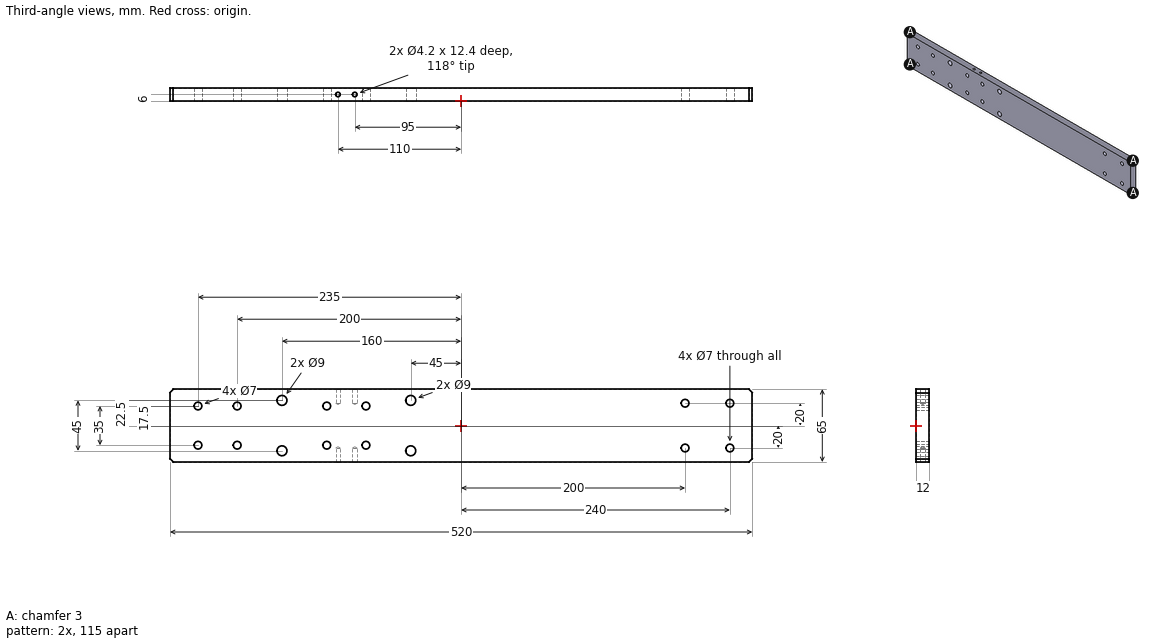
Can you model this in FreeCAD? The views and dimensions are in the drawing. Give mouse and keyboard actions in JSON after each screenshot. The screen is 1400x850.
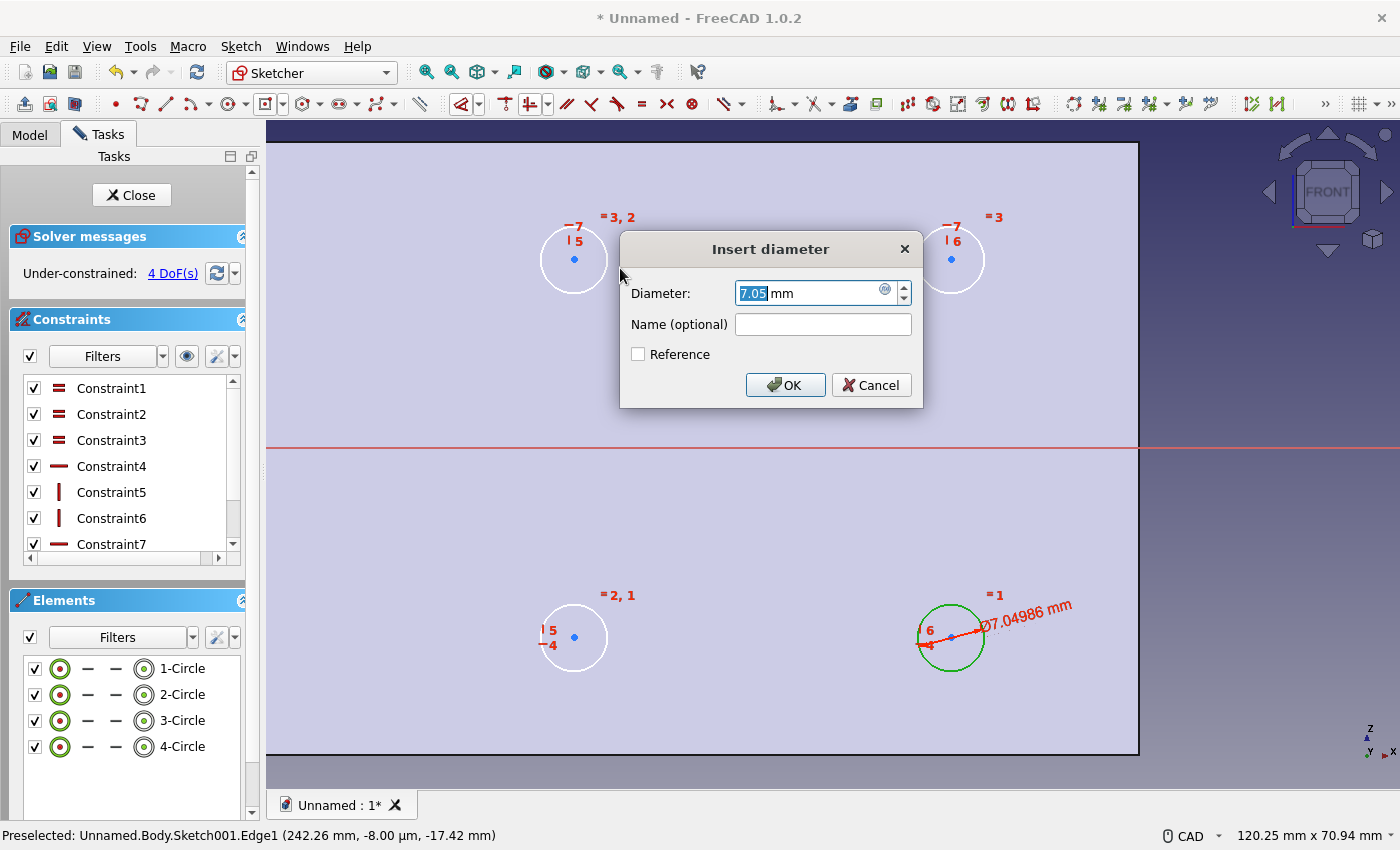
{"action": "type", "text": "7"}
{"action": "key", "text": "Return"}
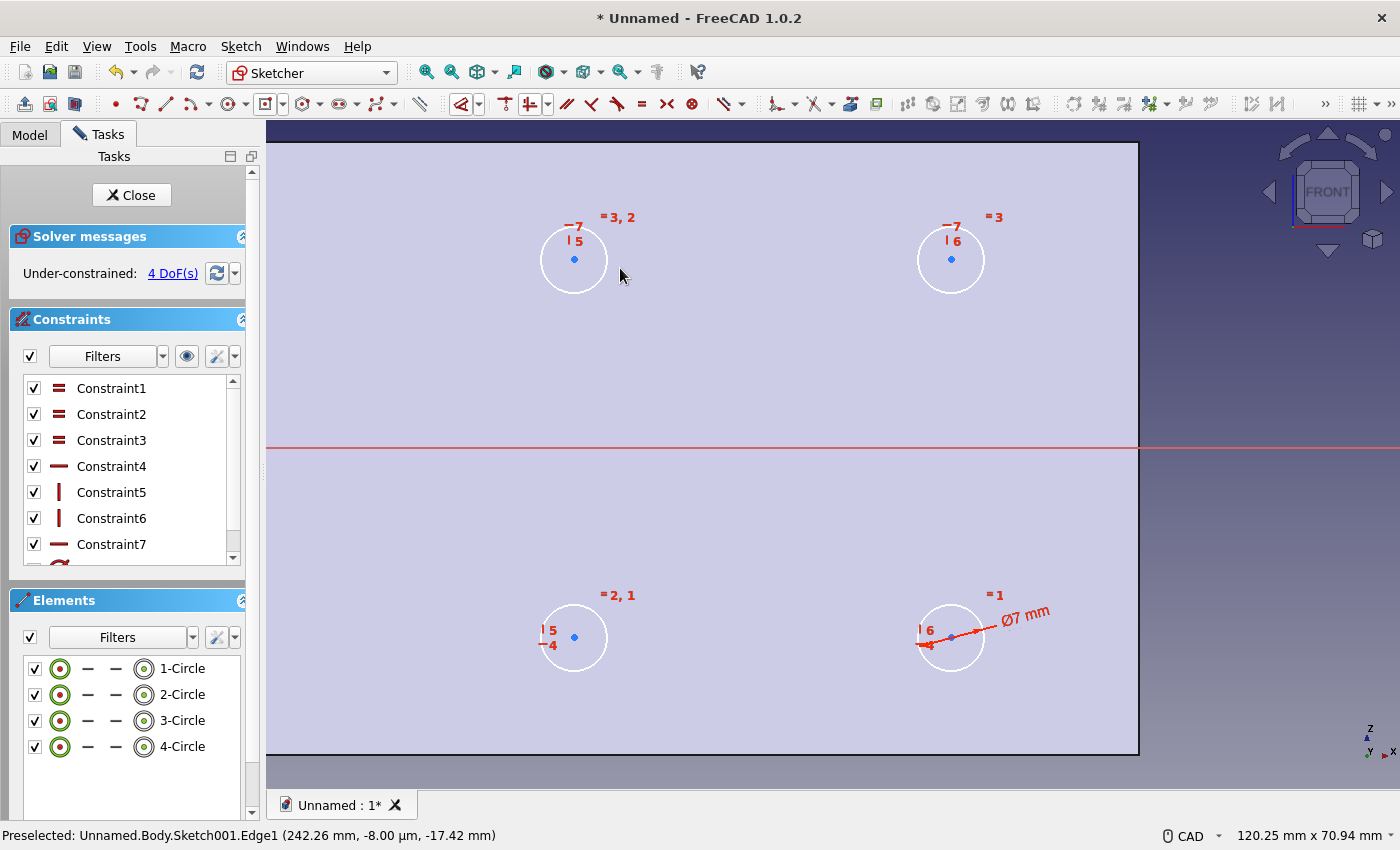
{"action": "left_click", "coordinate": [951, 638]}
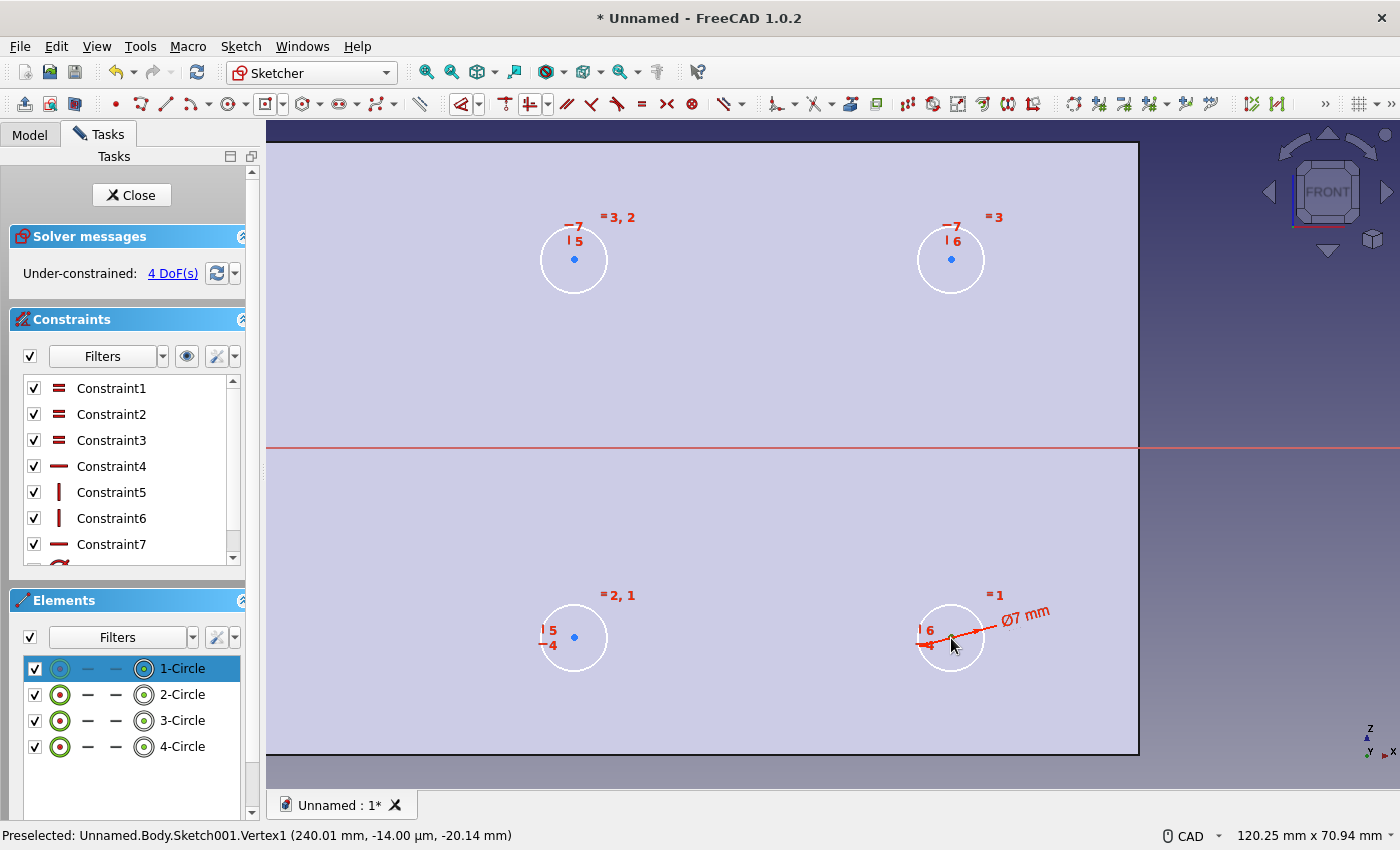
{"action": "key", "text": "i"}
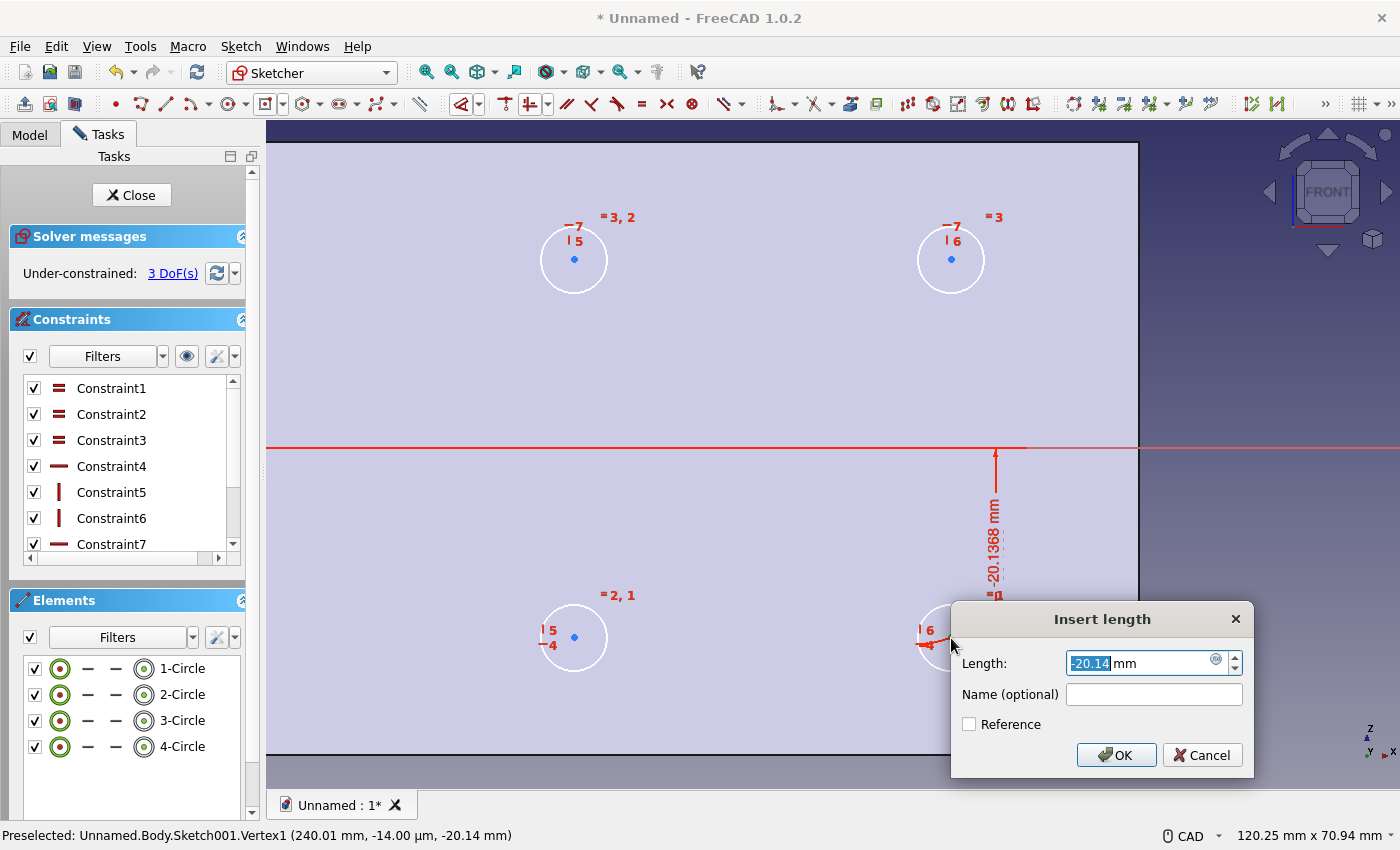
{"action": "type", "text": "-20"}
{"action": "key", "text": "Return"}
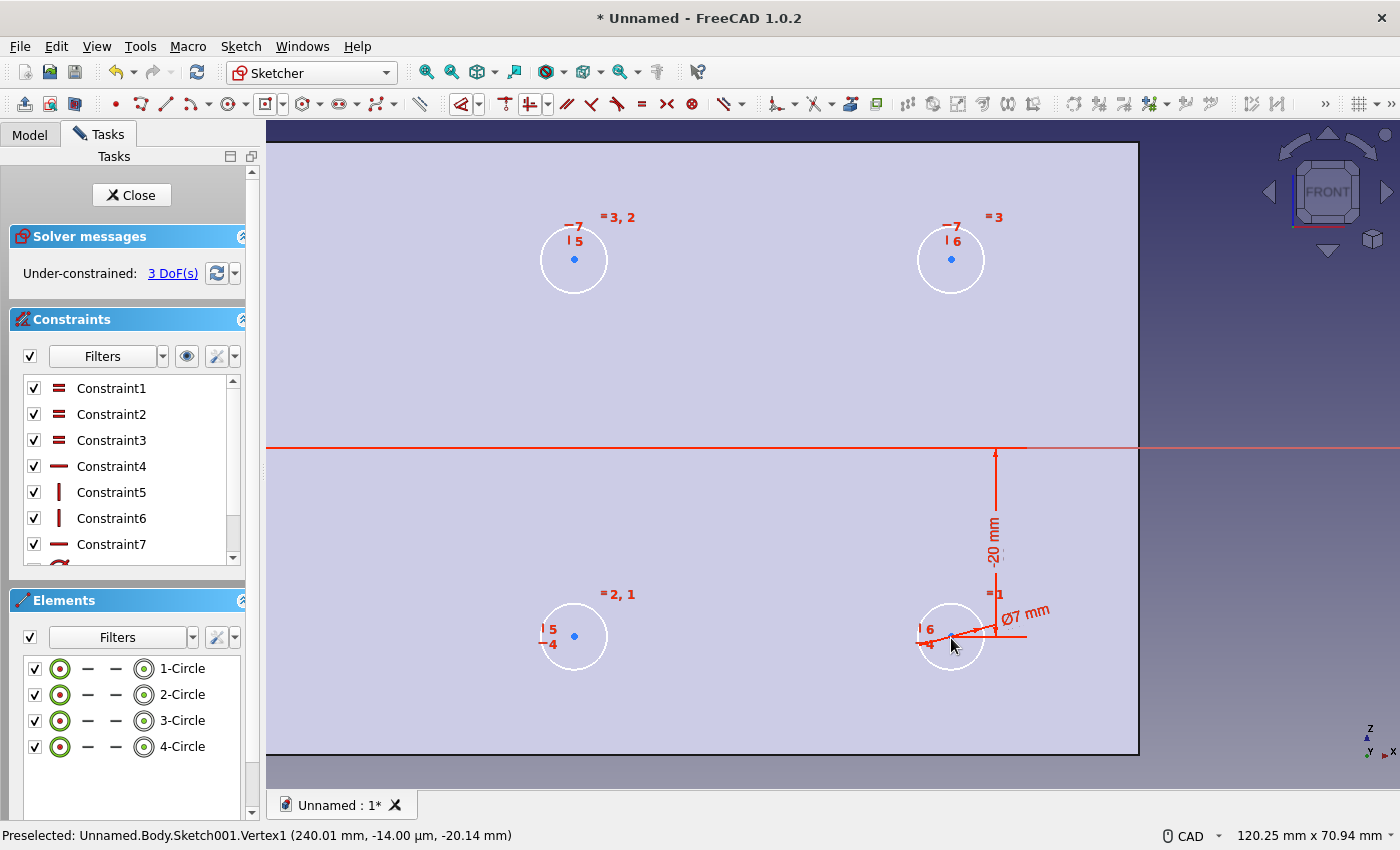
{"action": "left_click", "coordinate": [574, 260]}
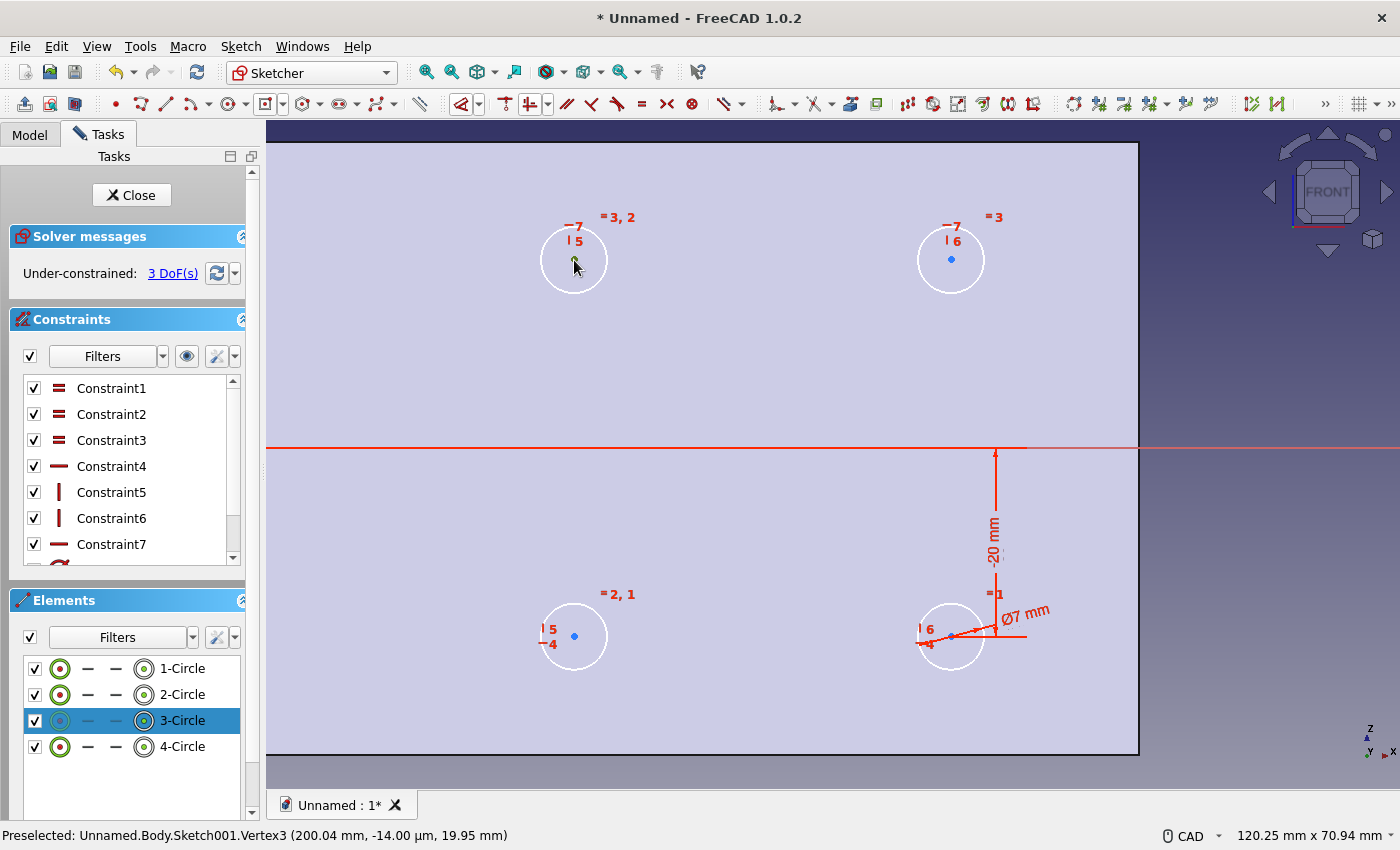
{"action": "left_click", "coordinate": [478, 104]}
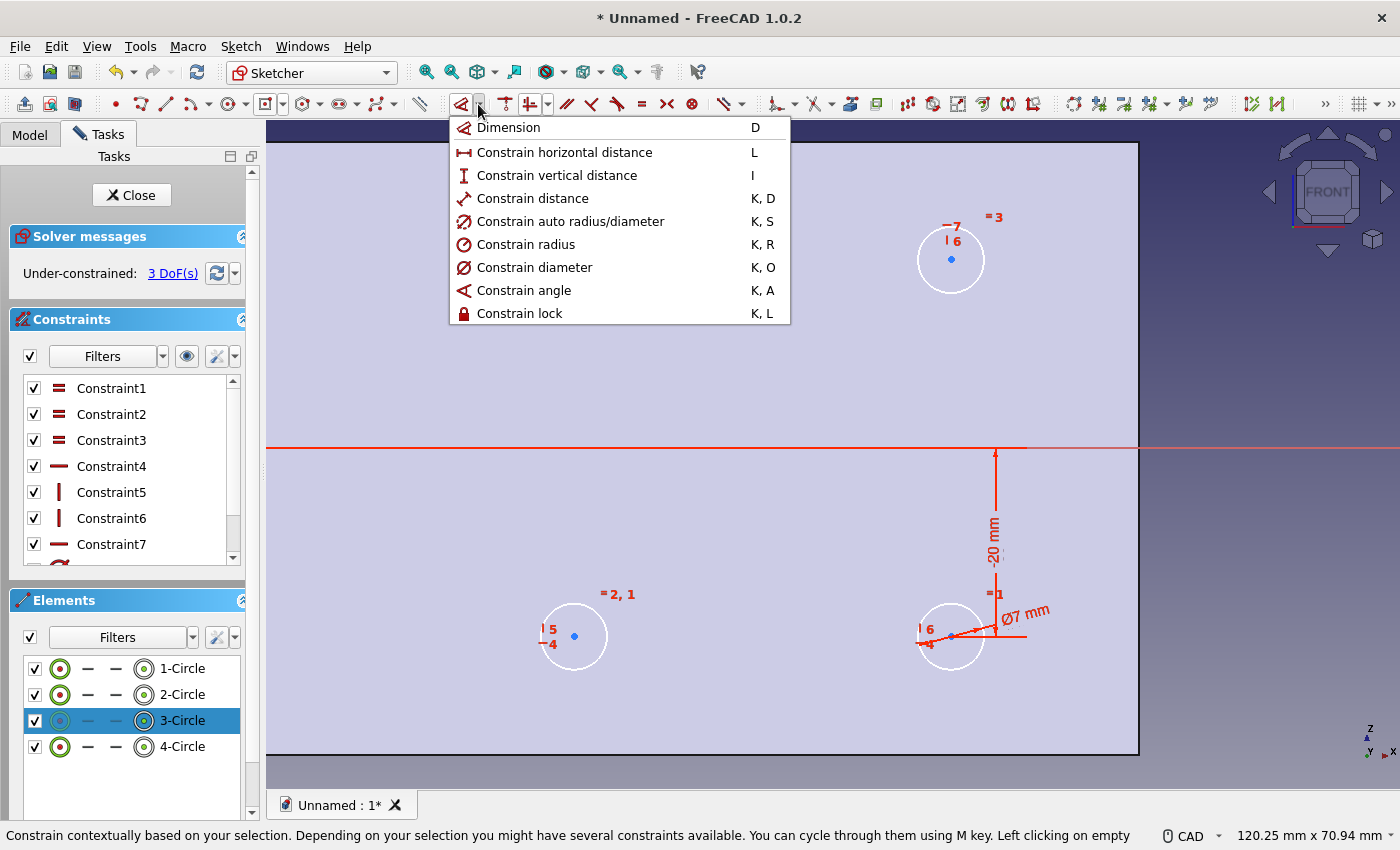
{"action": "left_click", "coordinate": [620, 176]}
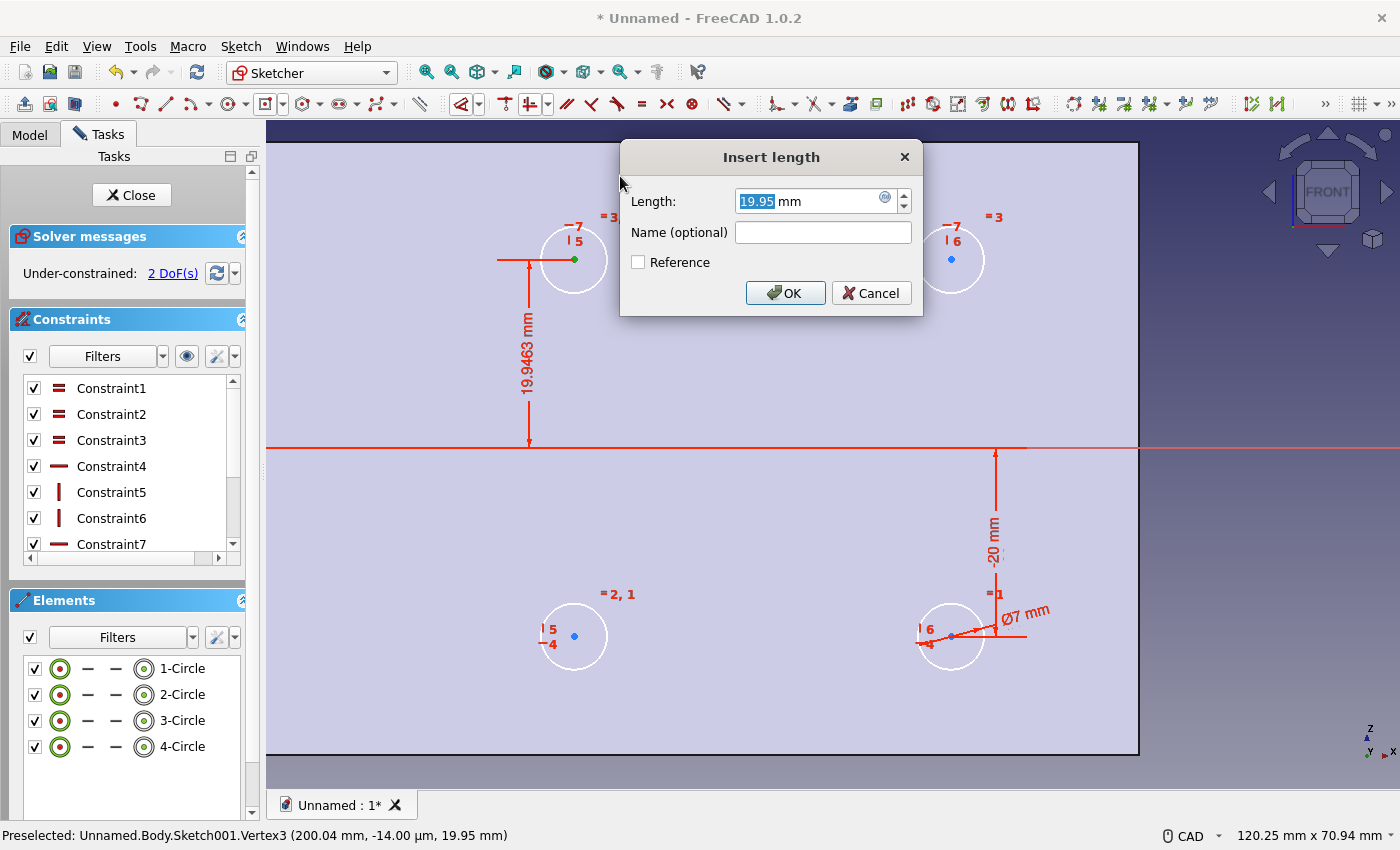
{"action": "type", "text": "20"}
{"action": "key", "text": "Return"}